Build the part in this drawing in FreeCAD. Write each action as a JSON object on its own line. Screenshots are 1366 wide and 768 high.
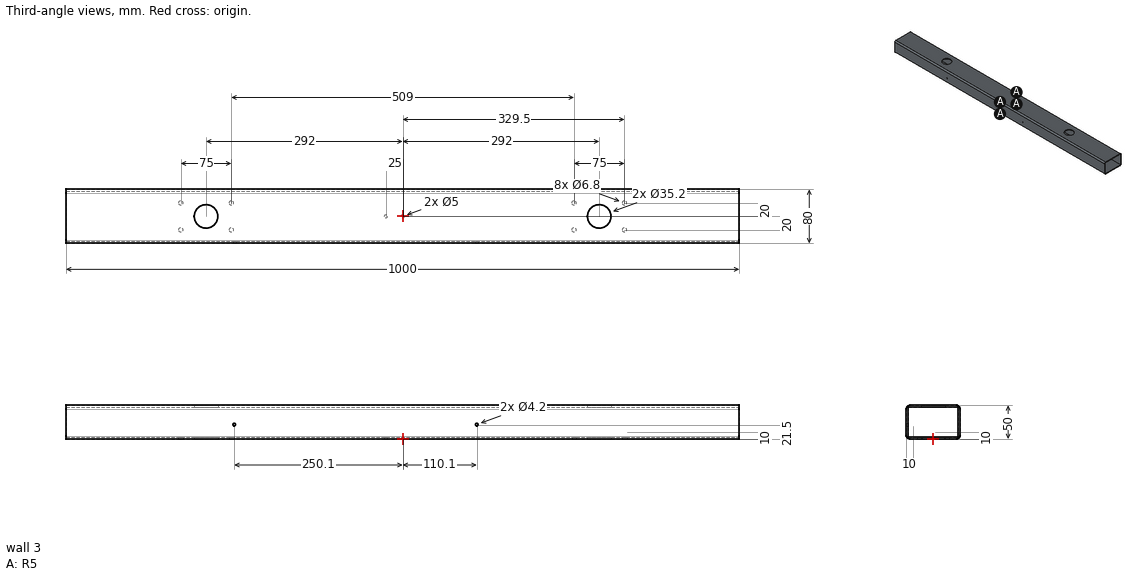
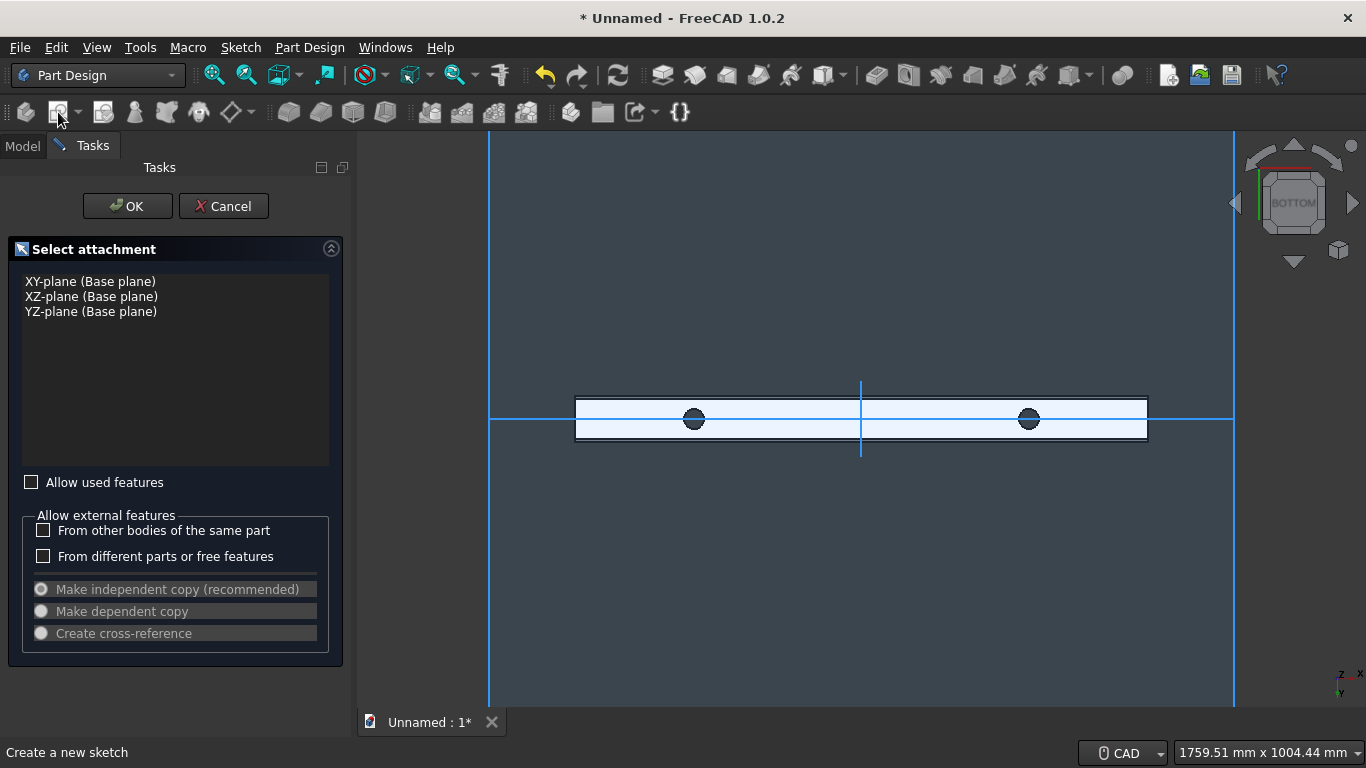
{"action": "left_click", "coordinate": [82, 282]}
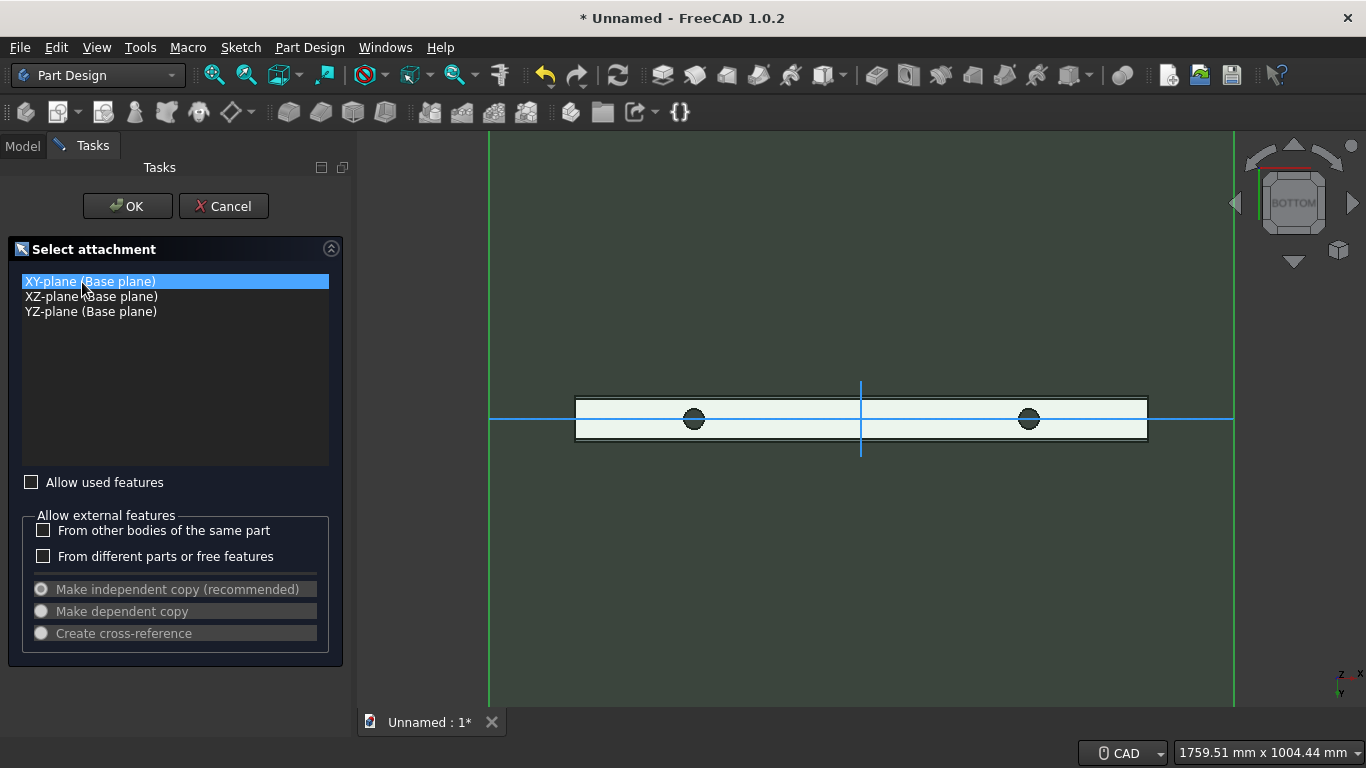
{"action": "left_click", "coordinate": [128, 206]}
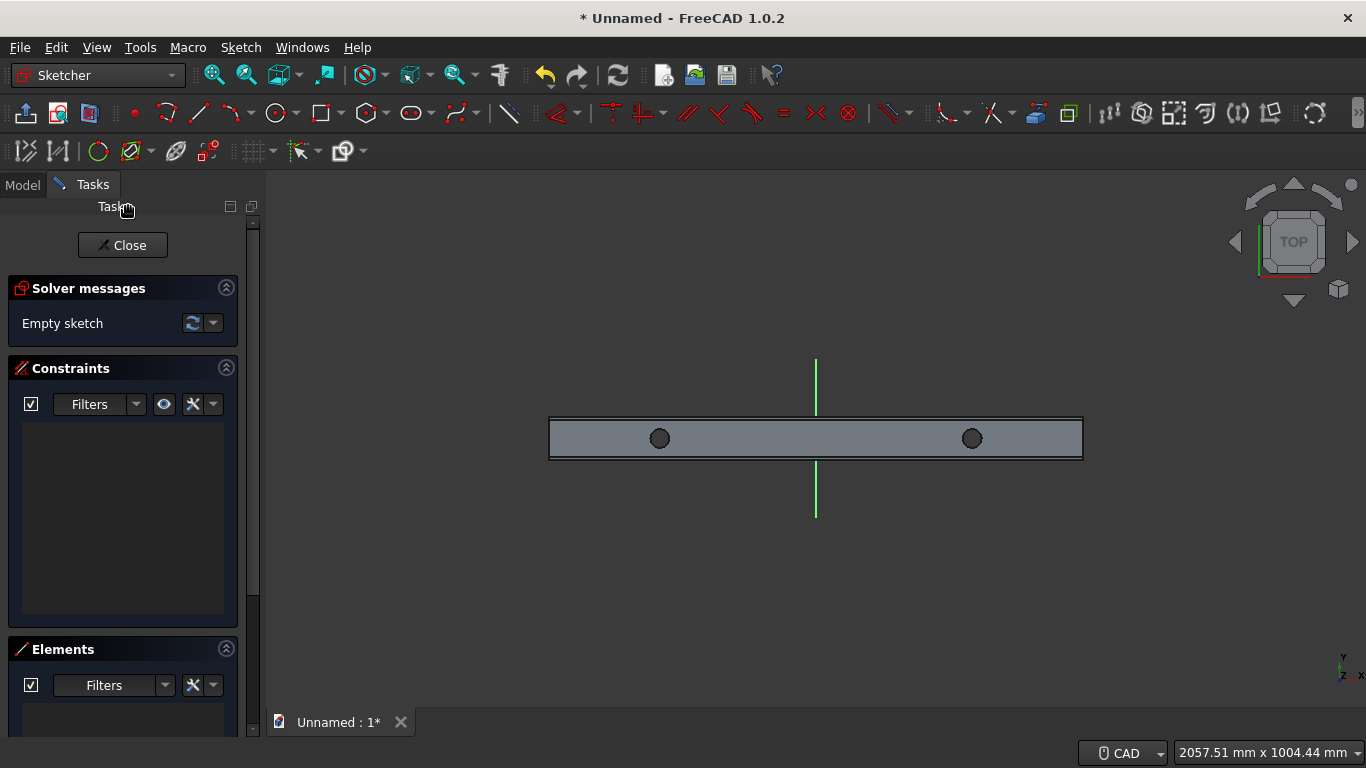
{"action": "left_click", "coordinate": [90, 114]}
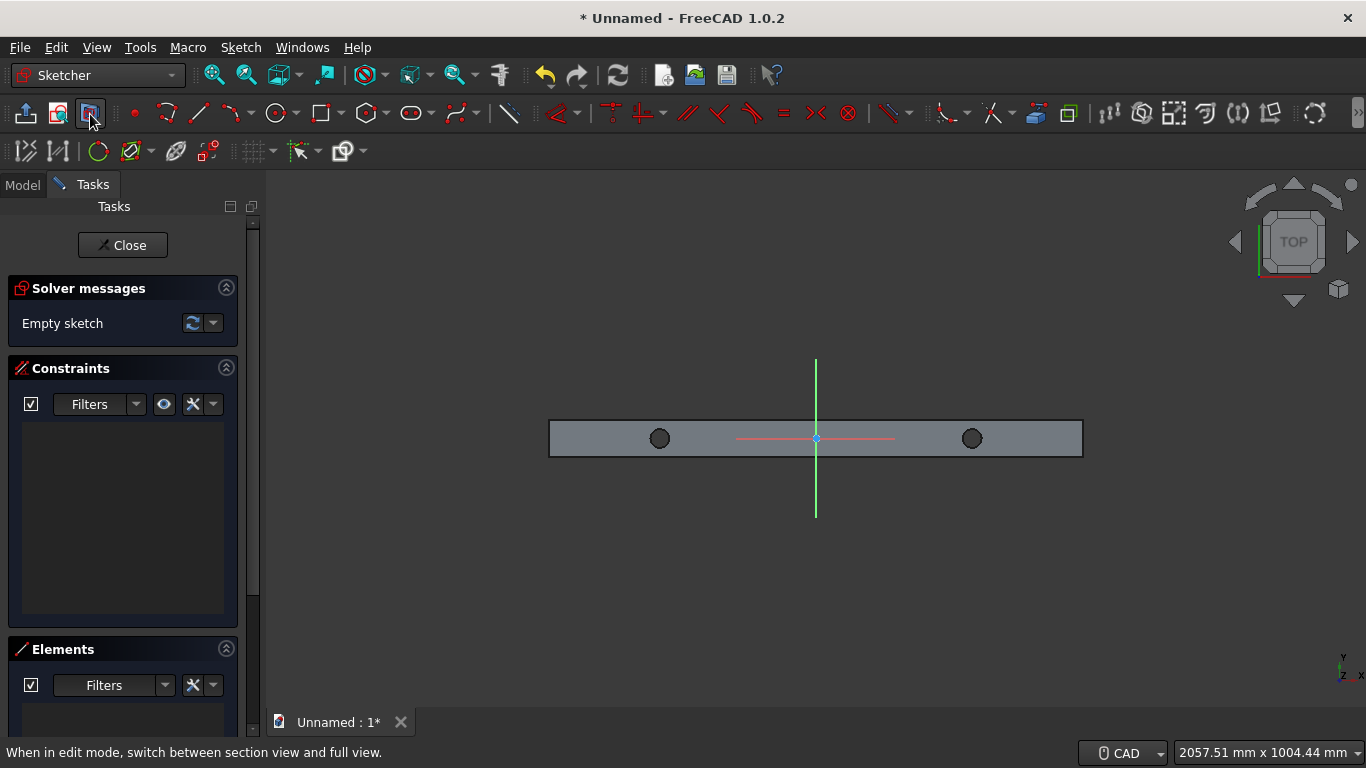
{"action": "scroll", "coordinate": [899, 438], "scroll_direction": "up", "scroll_amount": 3}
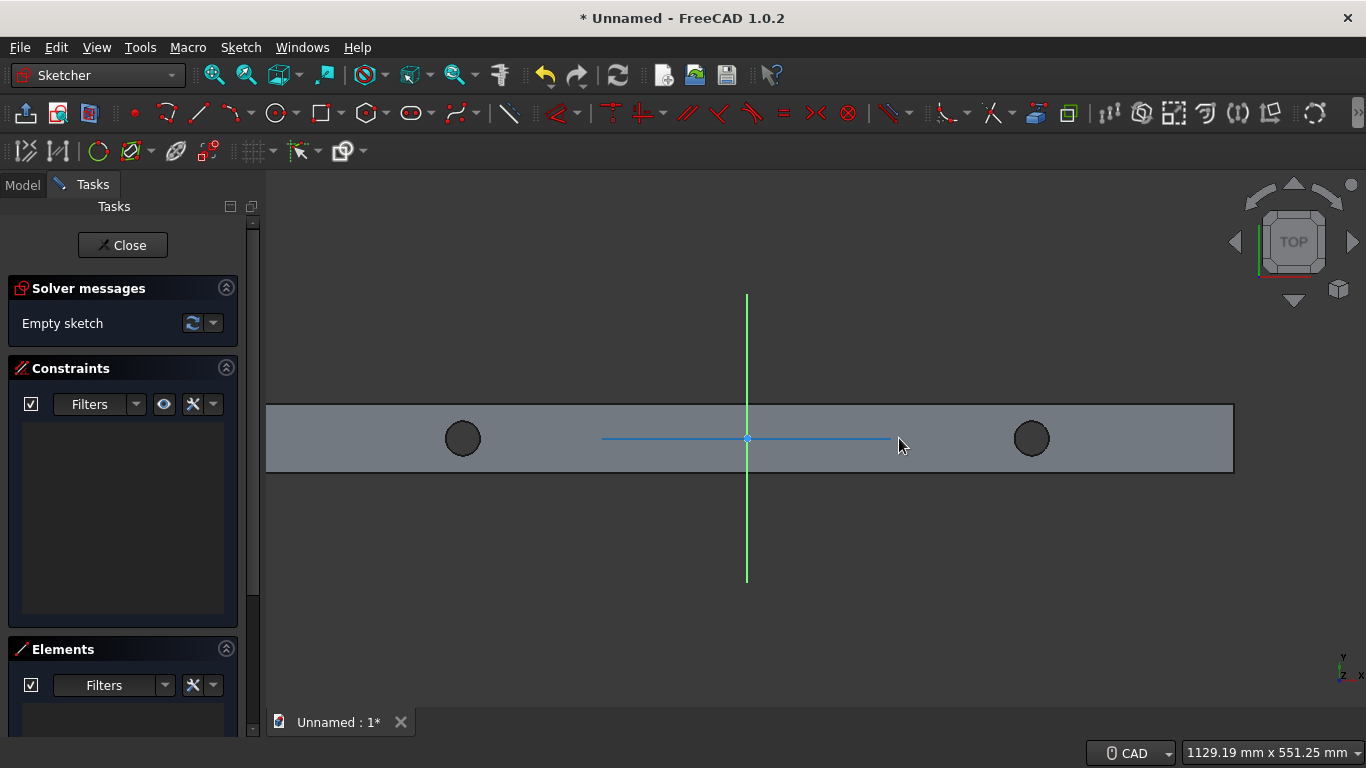
{"action": "left_click", "coordinate": [276, 114]}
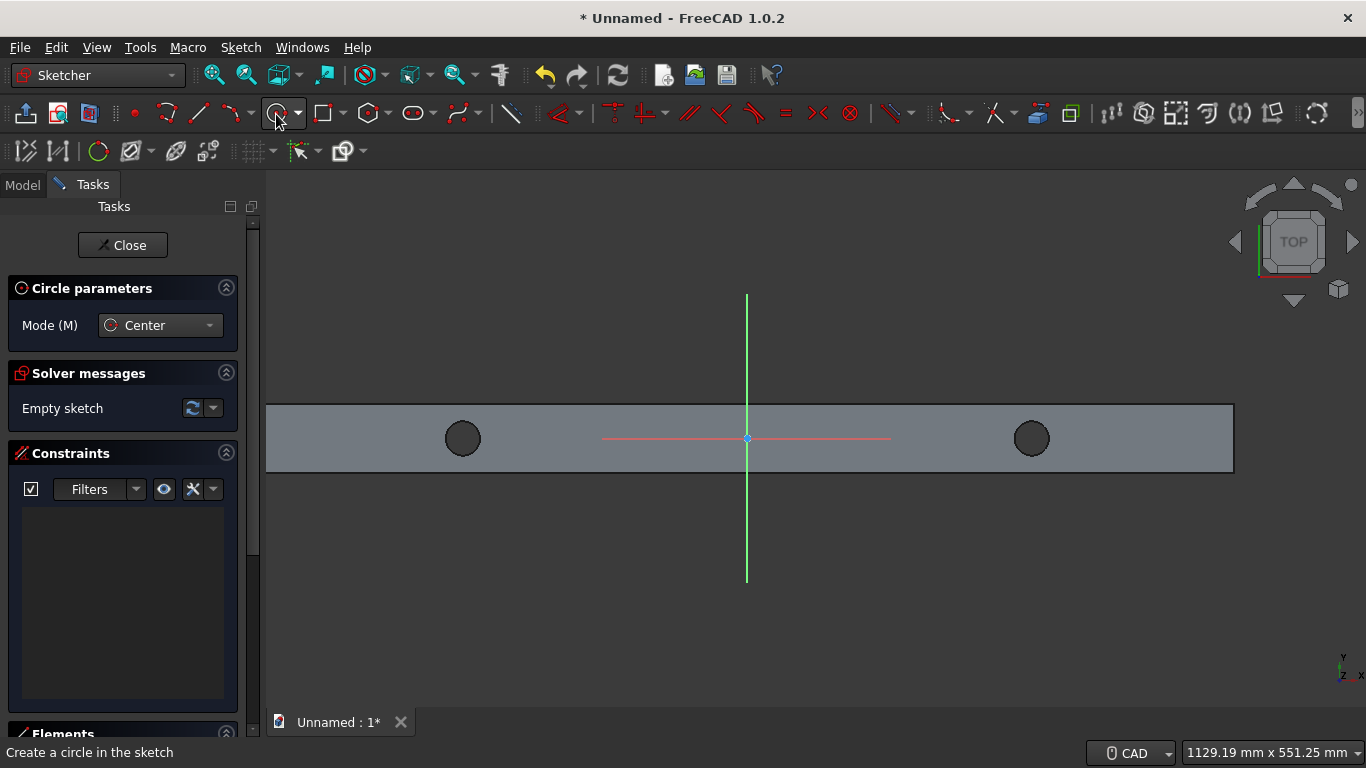
{"action": "scroll", "coordinate": [1068, 419], "scroll_direction": "up", "scroll_amount": 10}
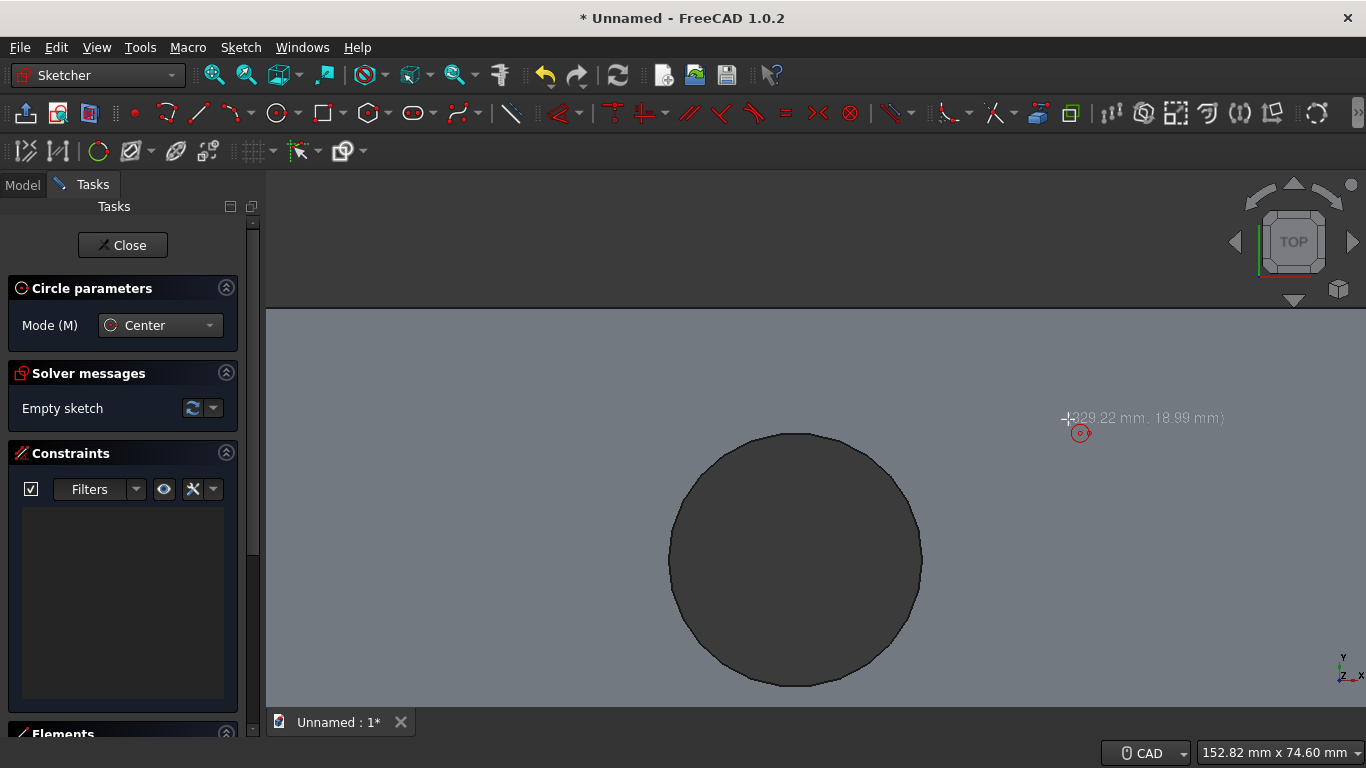
{"action": "scroll", "coordinate": [1069, 419], "scroll_direction": "down", "scroll_amount": 10}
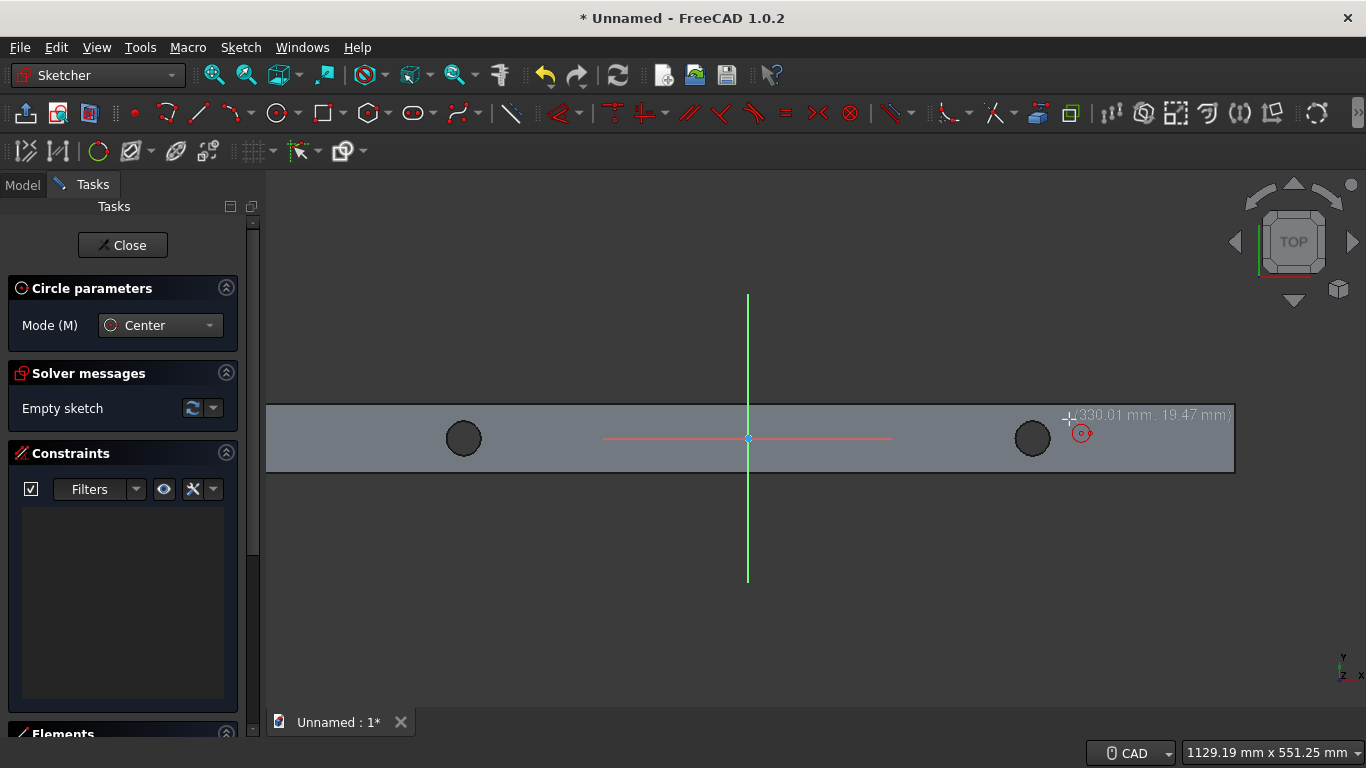
{"action": "left_click", "coordinate": [1069, 419]}
{"action": "mouse_move", "coordinate": [1071, 417]}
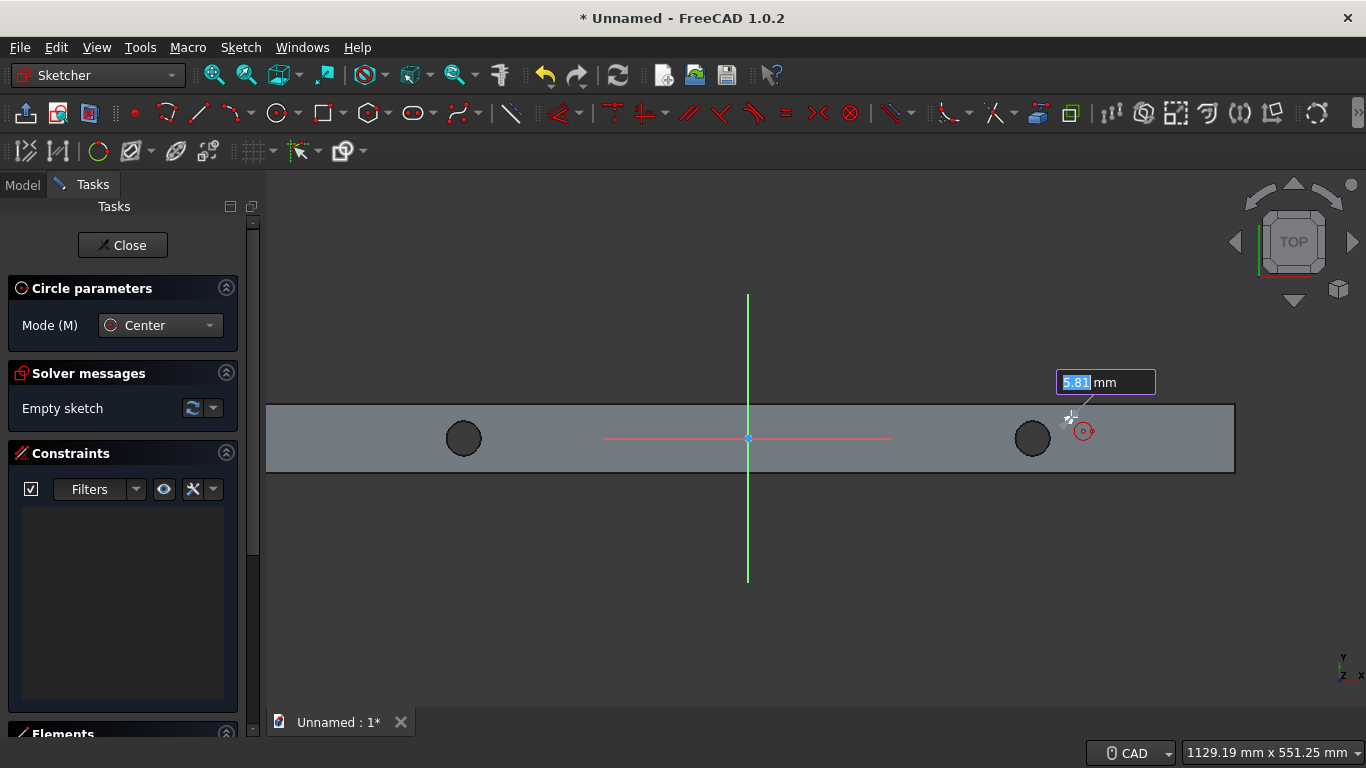
{"action": "type", "text": "6.8"}
{"action": "key", "text": "Return"}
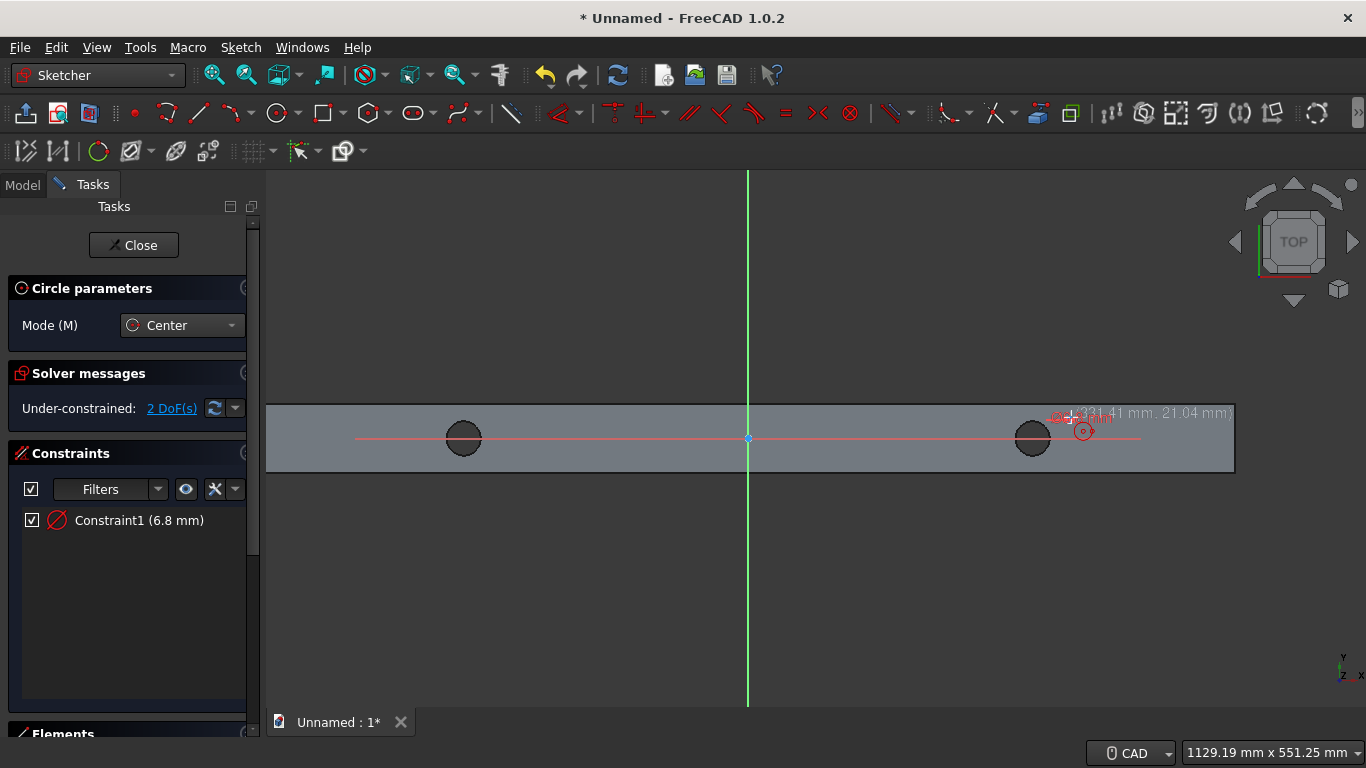
{"action": "scroll", "coordinate": [1069, 458], "scroll_direction": "up", "scroll_amount": 10}